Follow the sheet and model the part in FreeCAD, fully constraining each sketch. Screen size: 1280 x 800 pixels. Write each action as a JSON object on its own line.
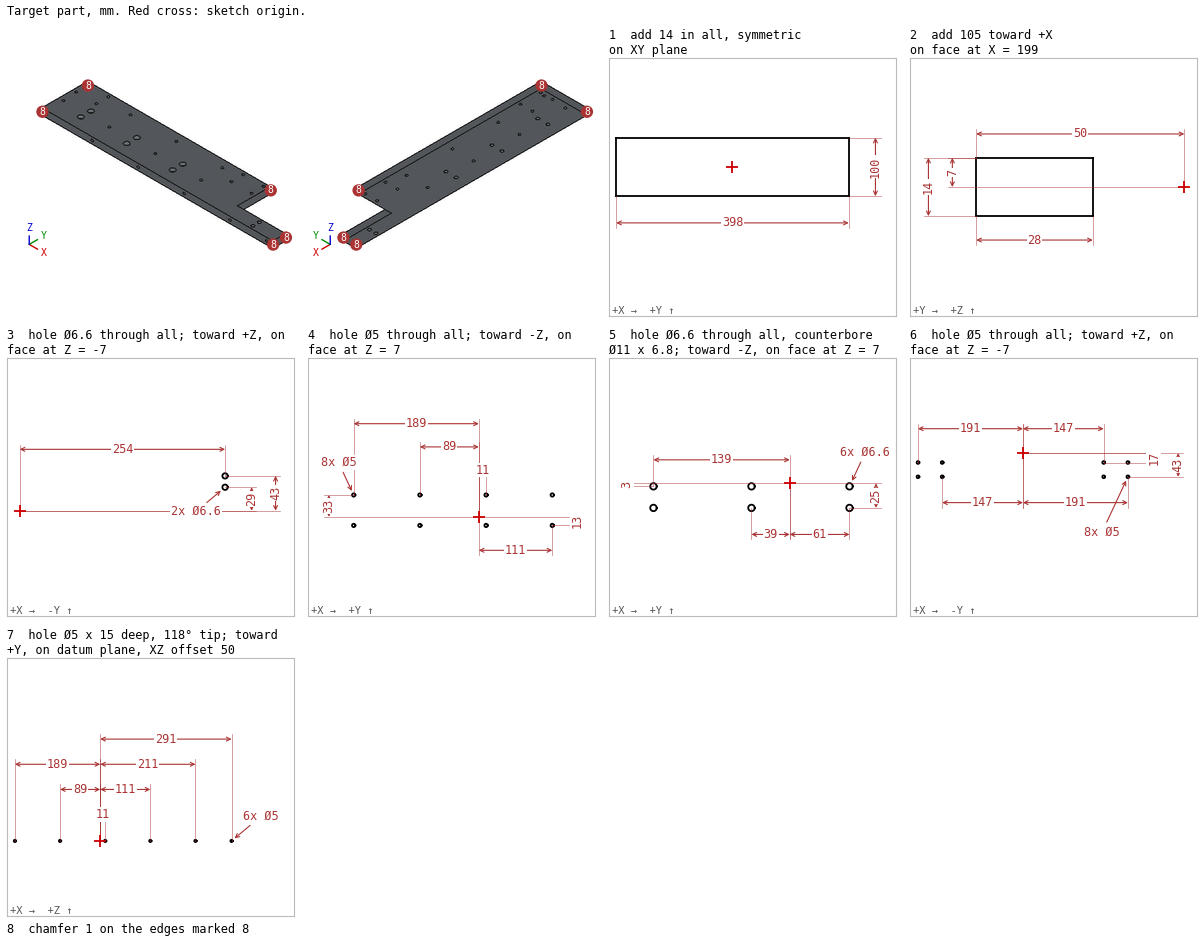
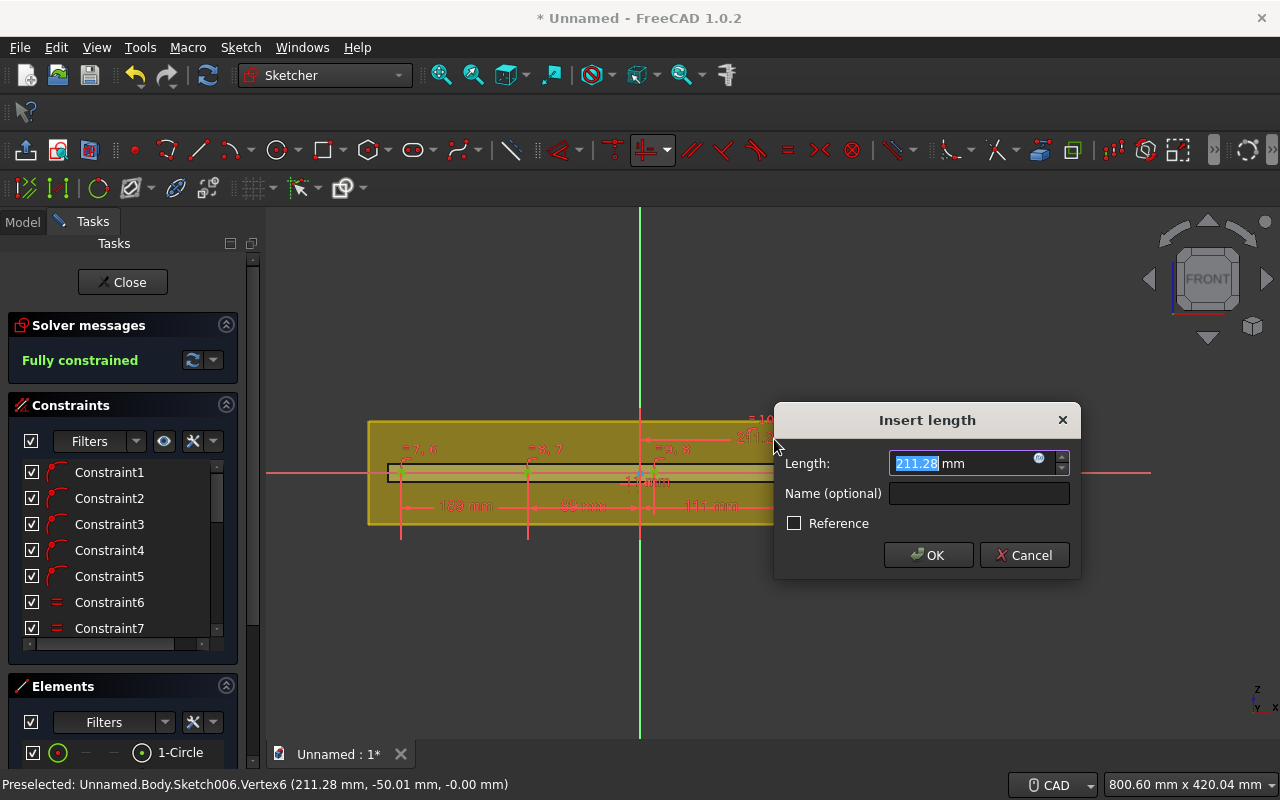
{"action": "type", "text": "211"}
{"action": "key", "text": "Return"}
{"action": "key", "text": "Escape"}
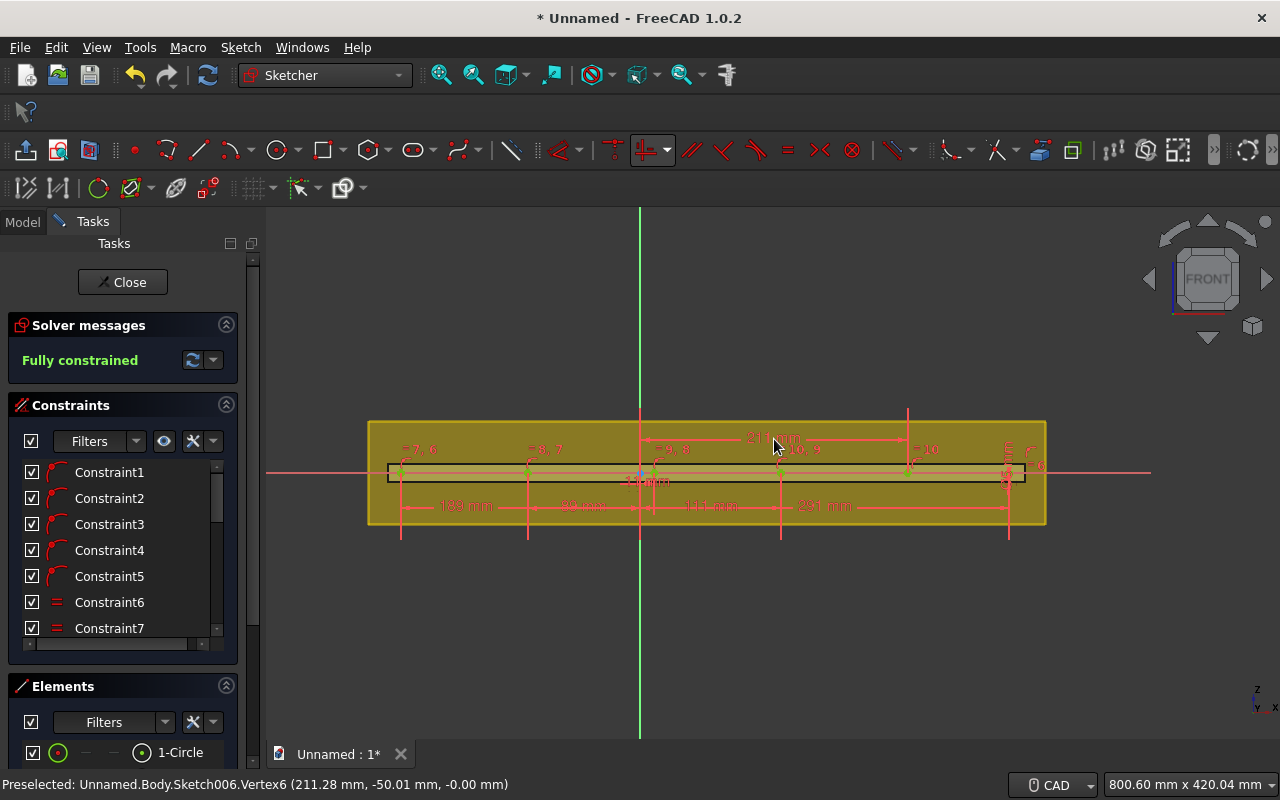
{"action": "left_click", "coordinate": [123, 282]}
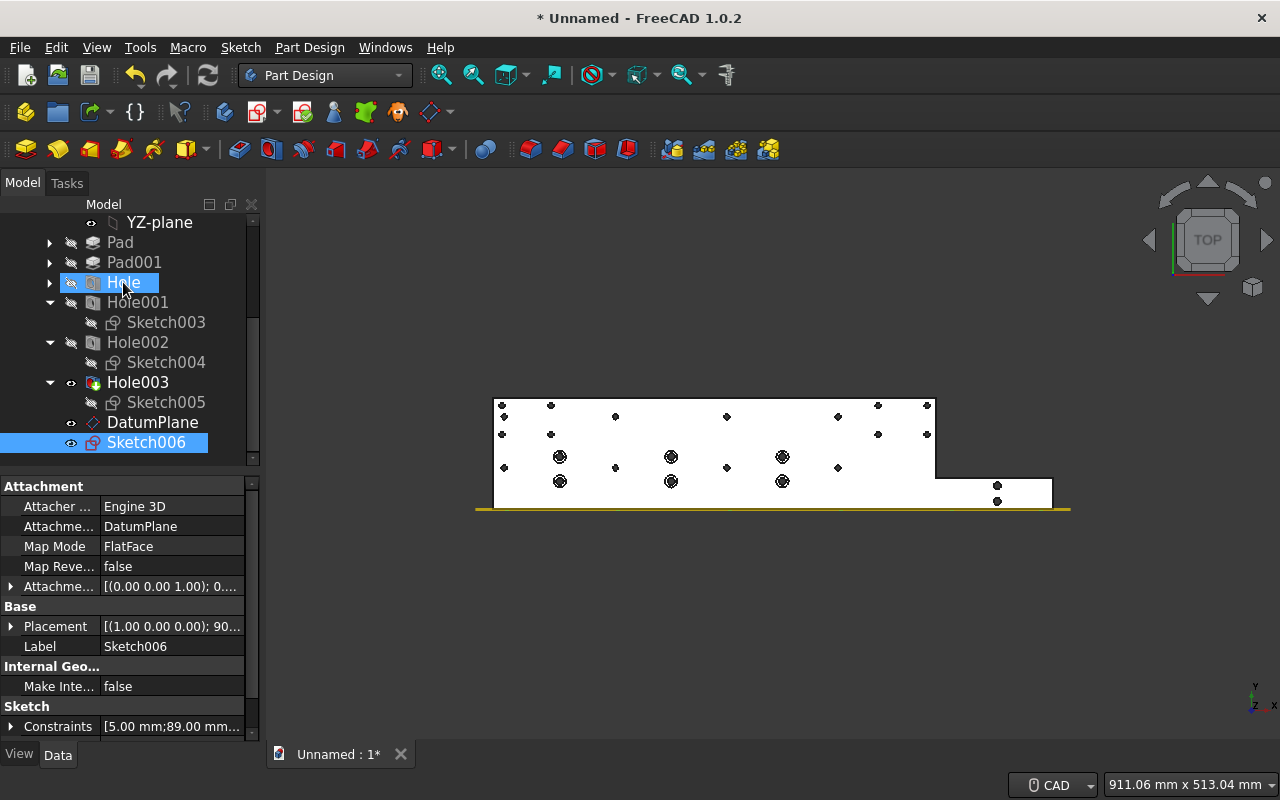
{"action": "left_click", "coordinate": [272, 150]}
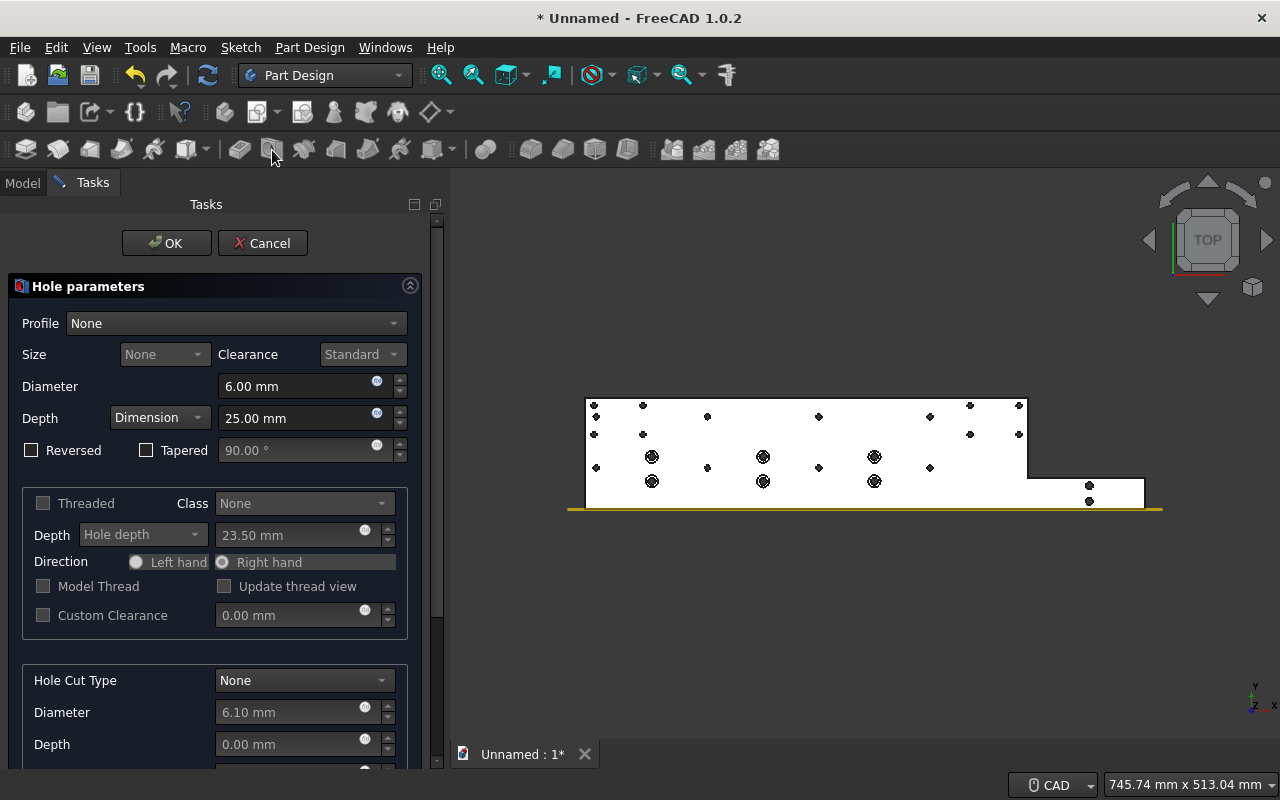
{"action": "triple_click", "coordinate": [305, 386]}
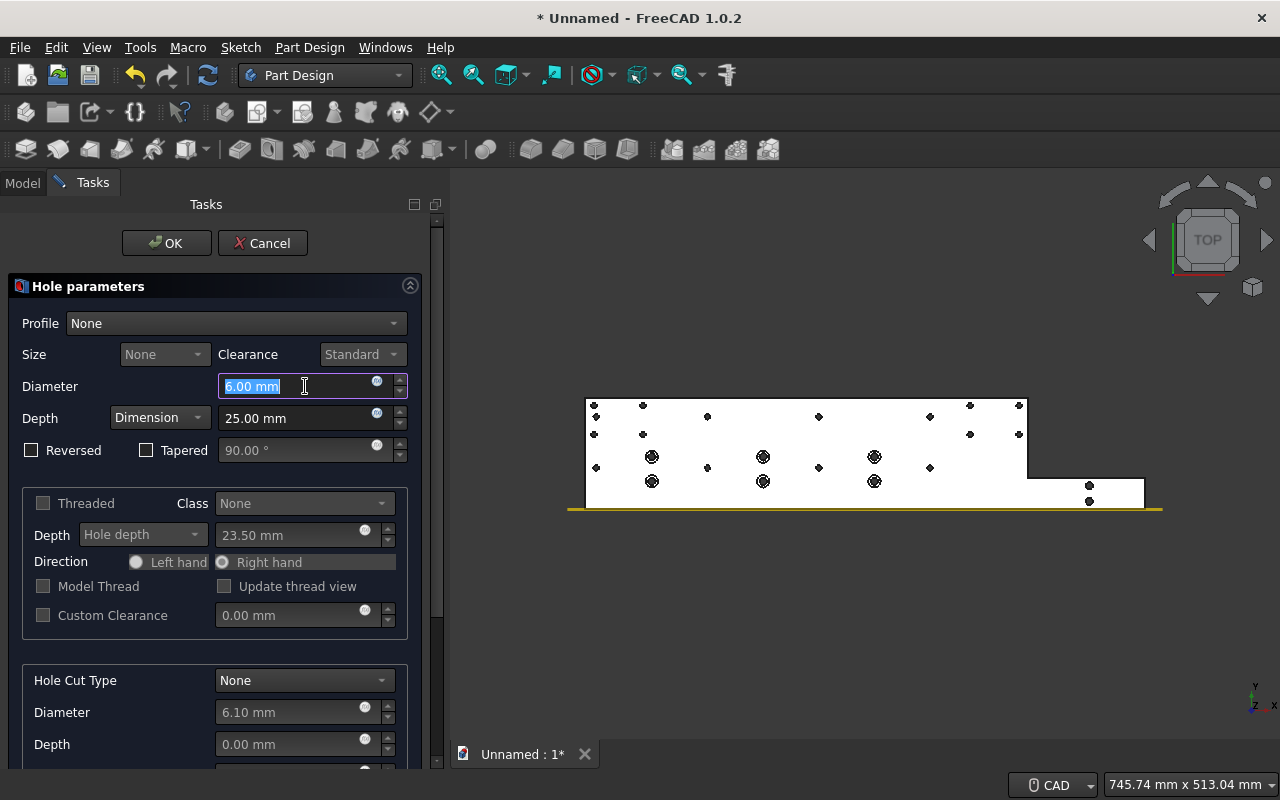
{"action": "type", "text": "5"}
{"action": "key", "text": "Tab"}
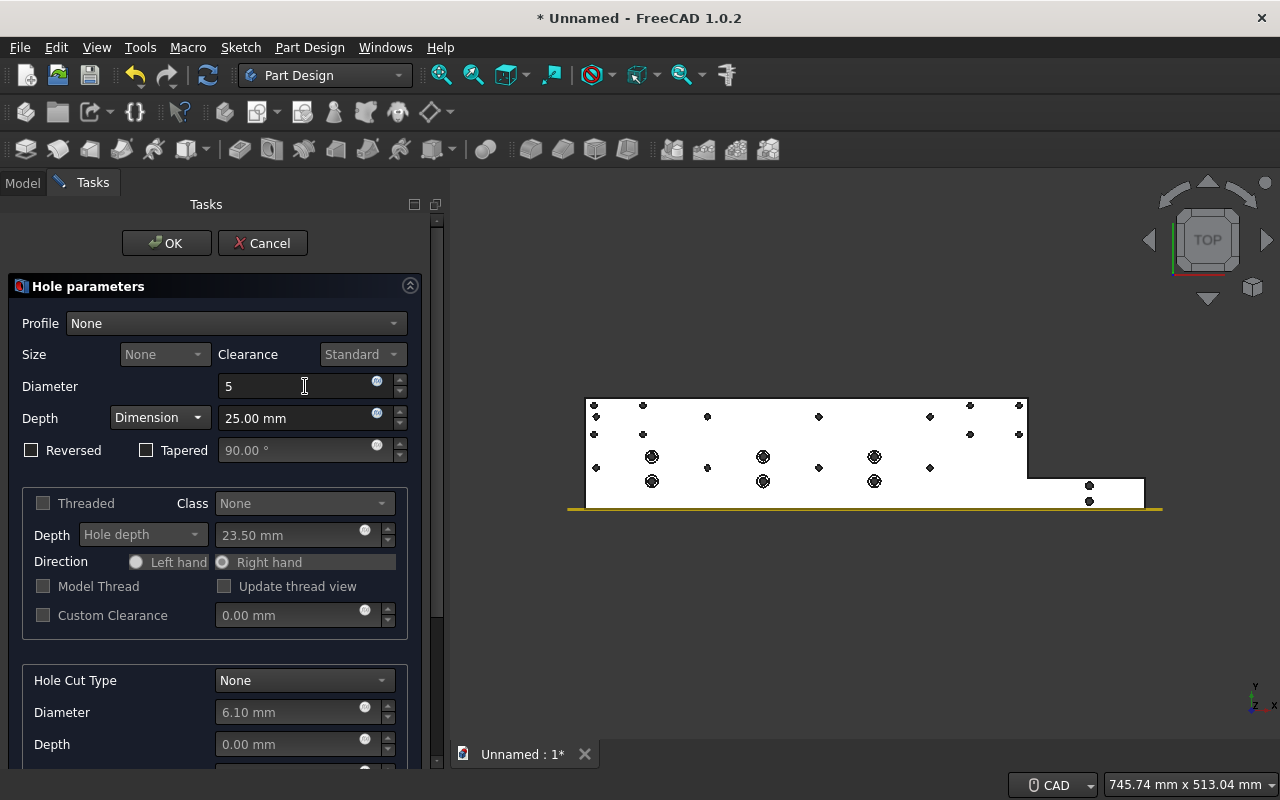
{"action": "triple_click", "coordinate": [305, 418]}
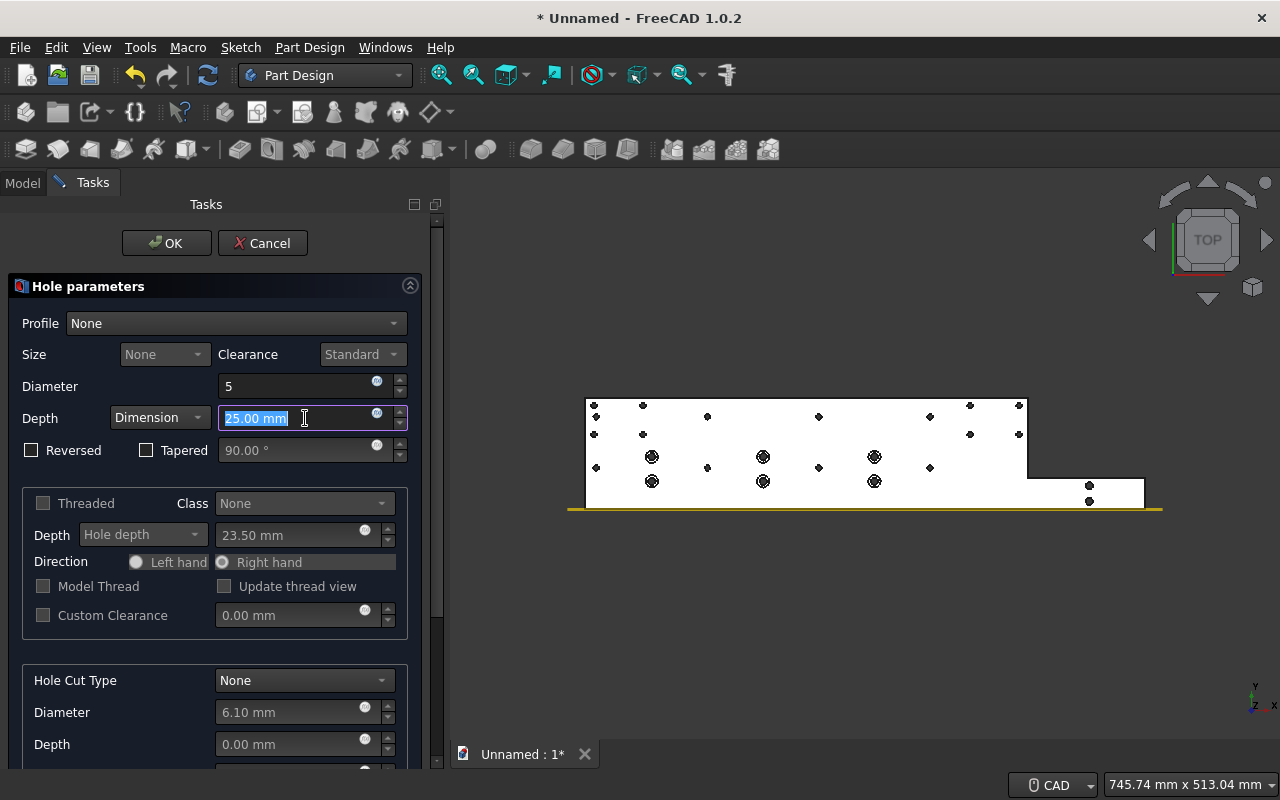
{"action": "type", "text": "15"}
{"action": "key", "text": "Tab"}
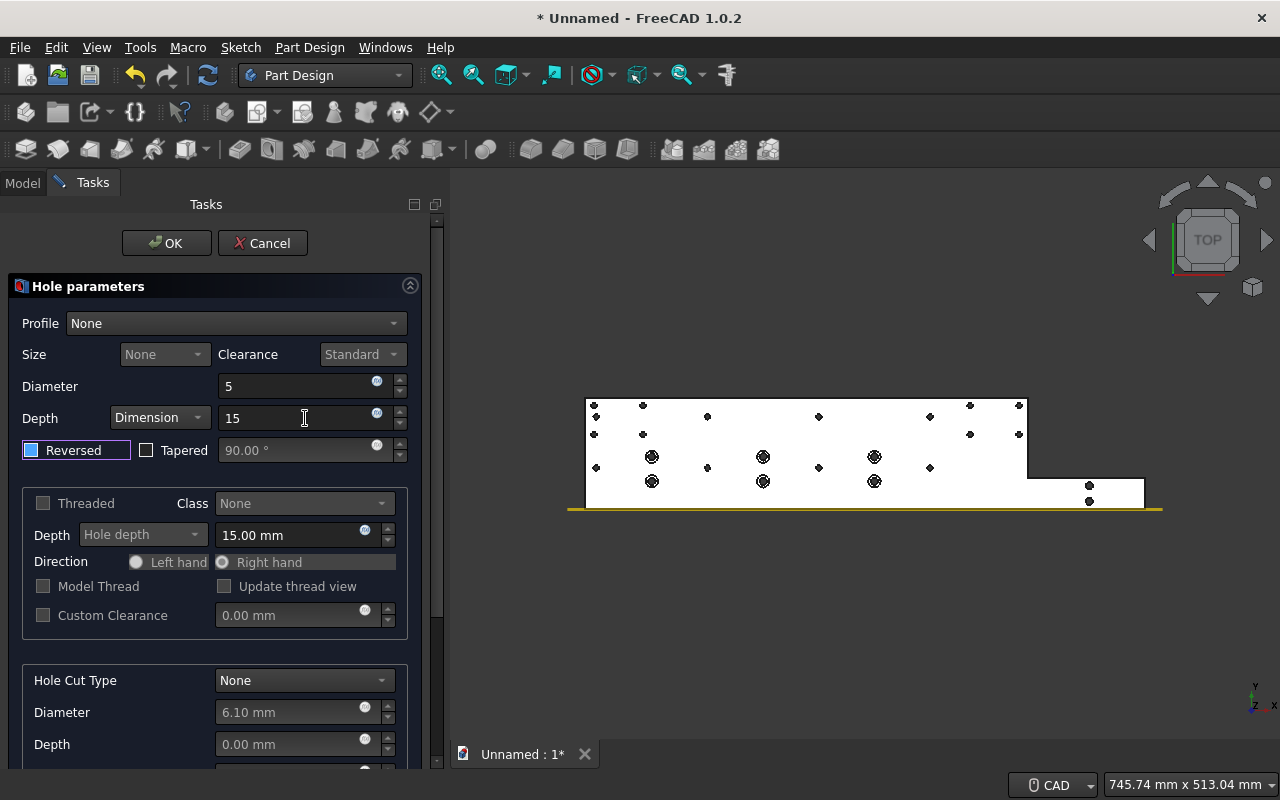
{"action": "left_click", "coordinate": [167, 243]}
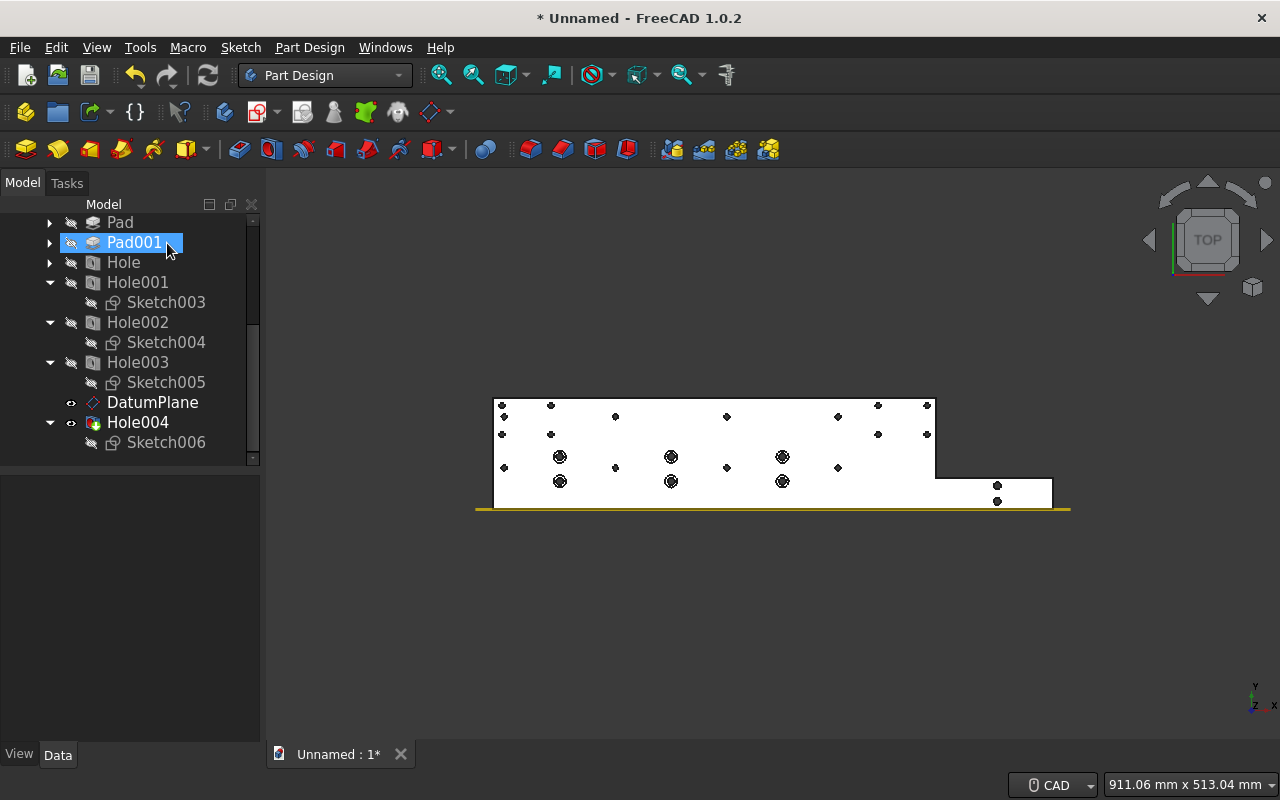
{"action": "left_click", "coordinate": [116, 403]}
{"action": "key", "text": "space"}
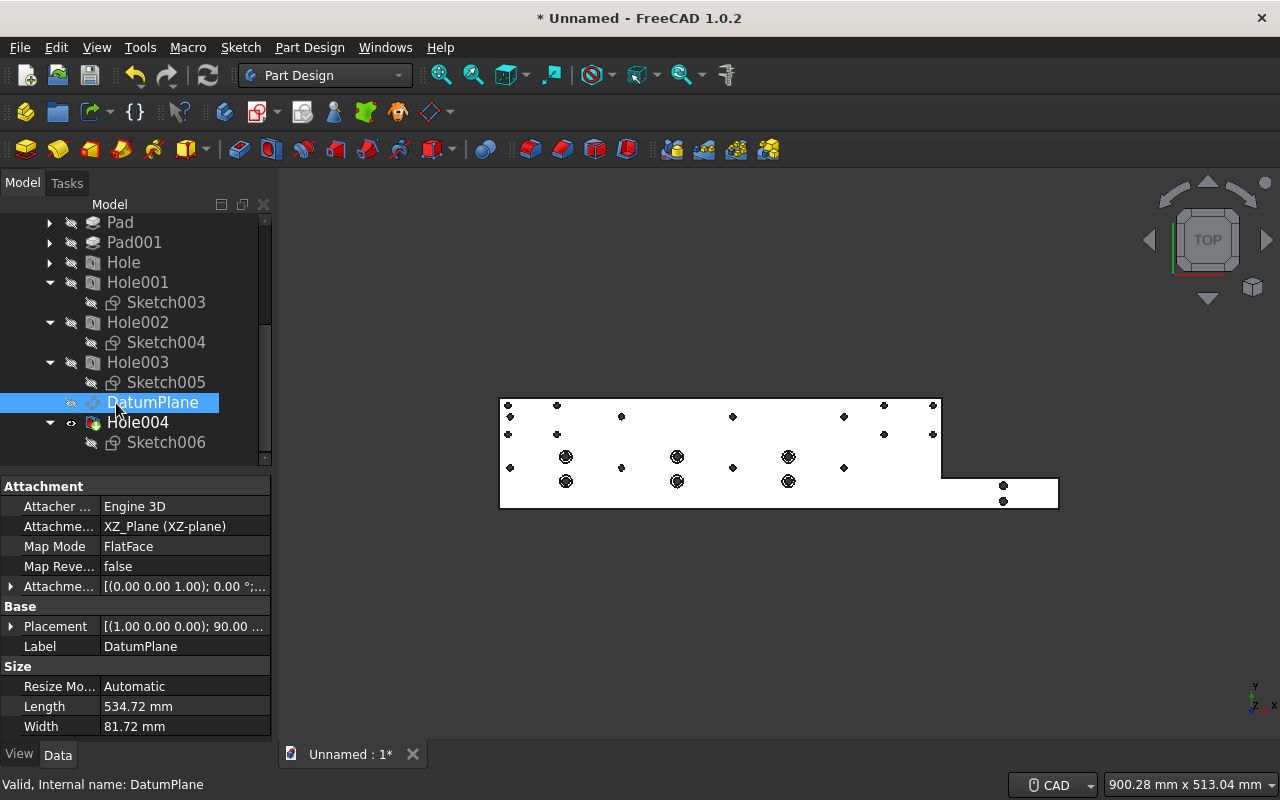
{"action": "scroll", "coordinate": [1059, 508], "scroll_direction": "up", "scroll_amount": 5}